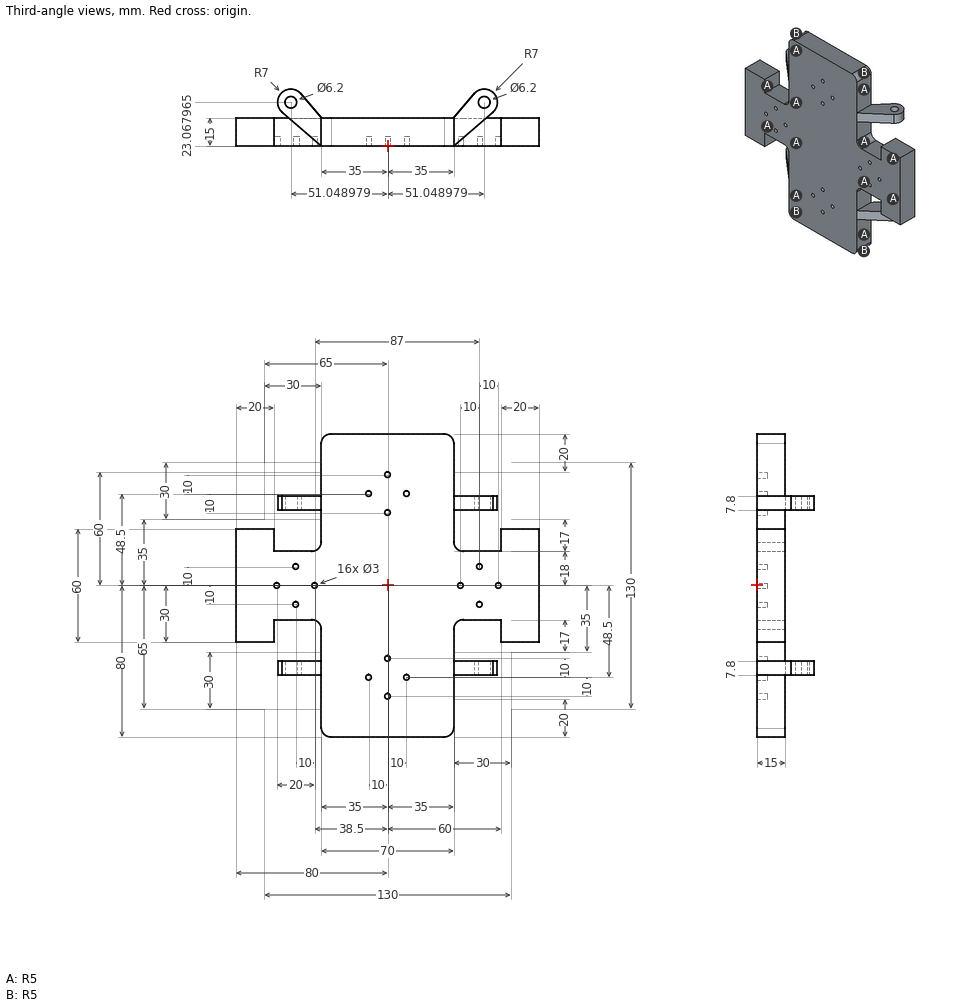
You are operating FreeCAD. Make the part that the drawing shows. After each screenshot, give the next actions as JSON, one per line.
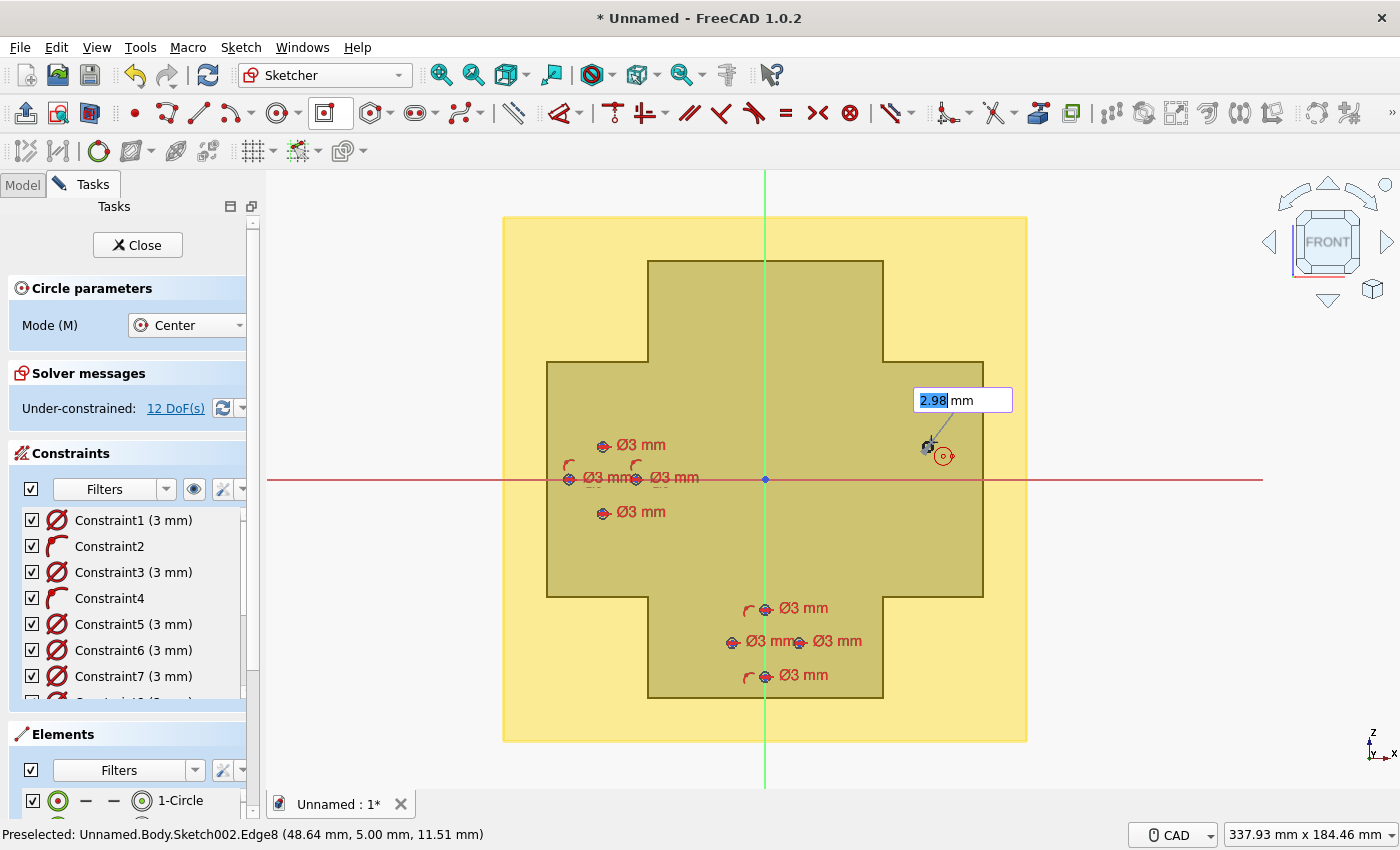
{"action": "type", "text": "3"}
{"action": "key", "text": "Return"}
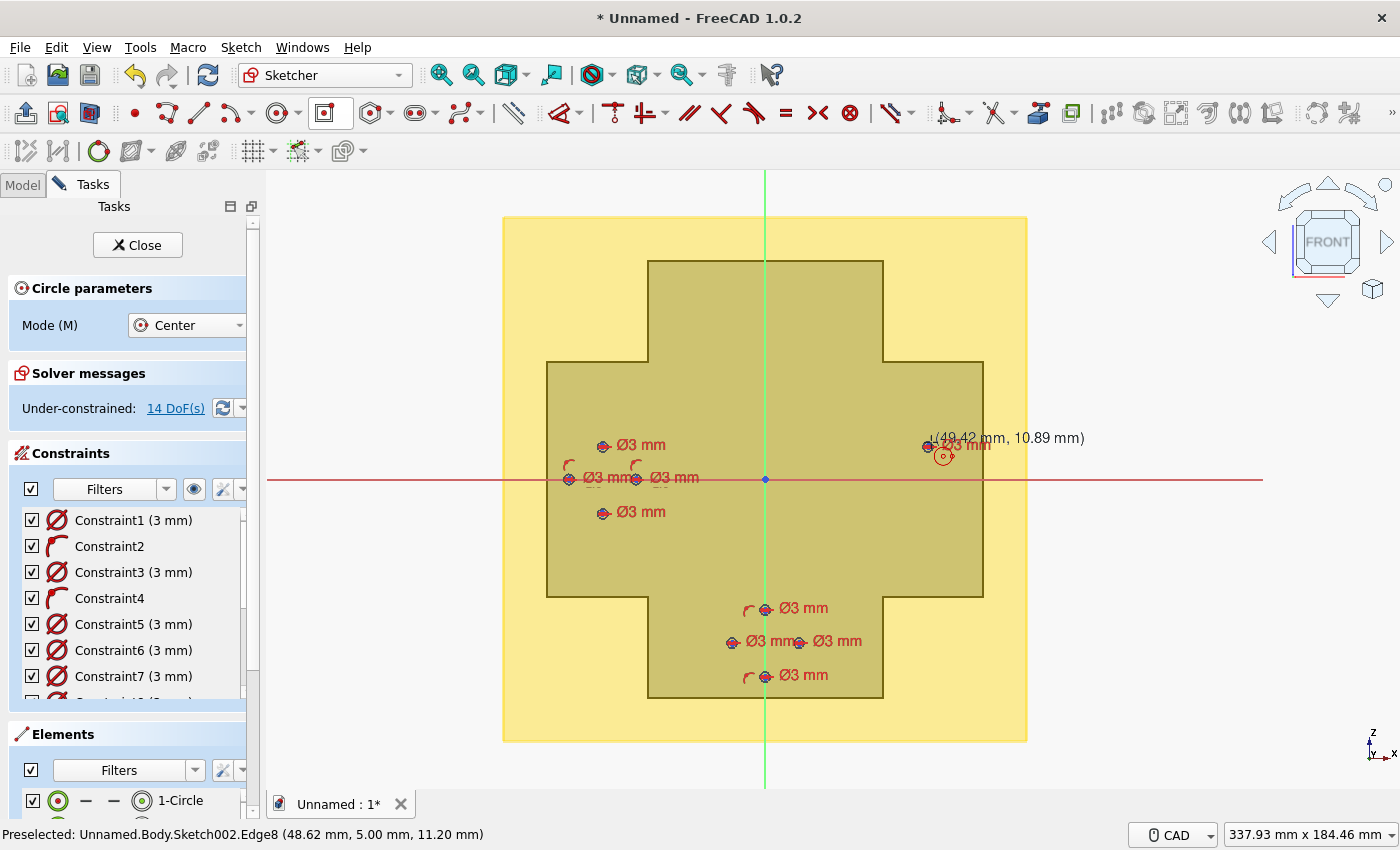
{"action": "scroll", "coordinate": [894, 480], "scroll_direction": "up", "scroll_amount": 8}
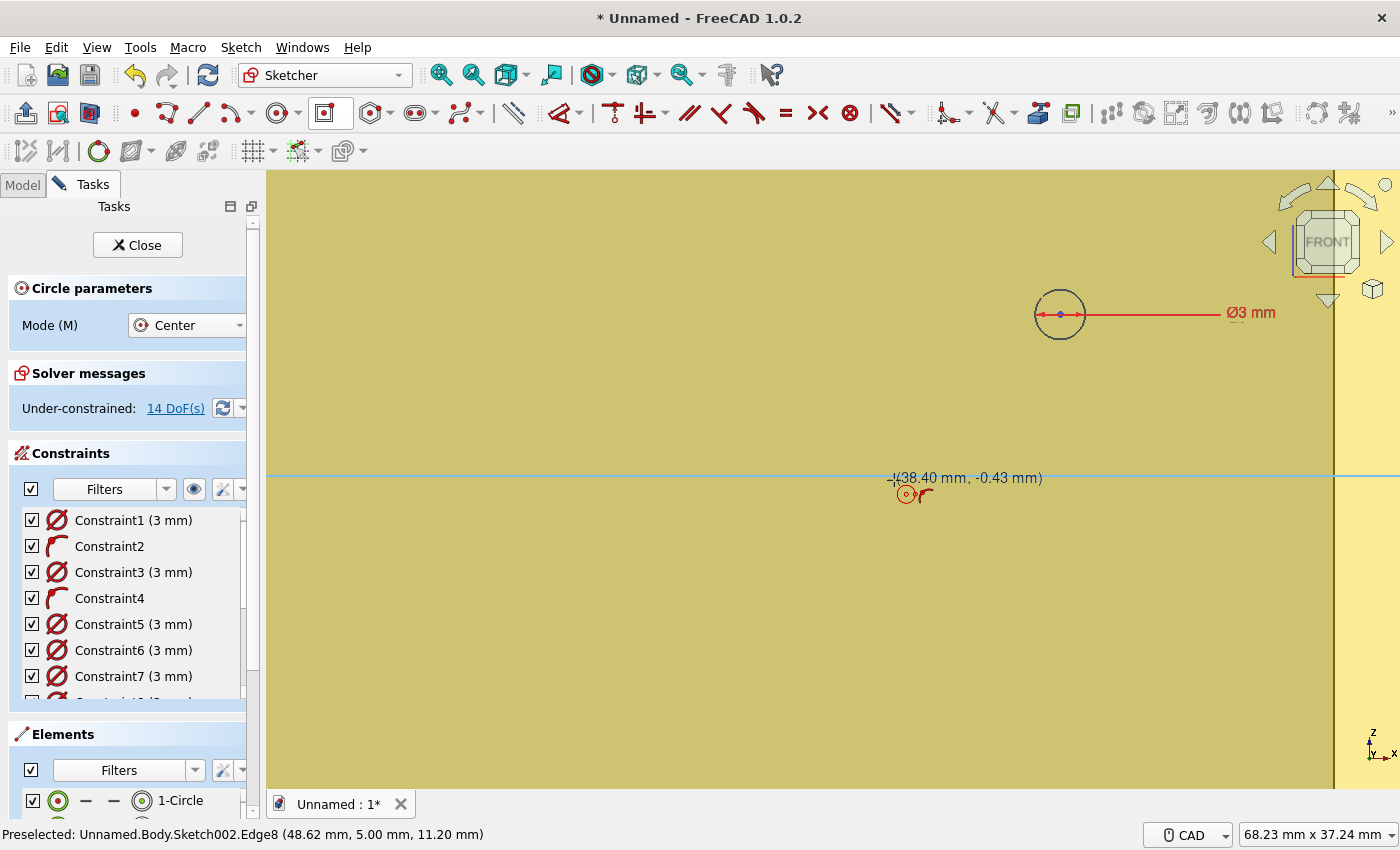
{"action": "scroll", "coordinate": [894, 480], "scroll_direction": "down", "scroll_amount": 8}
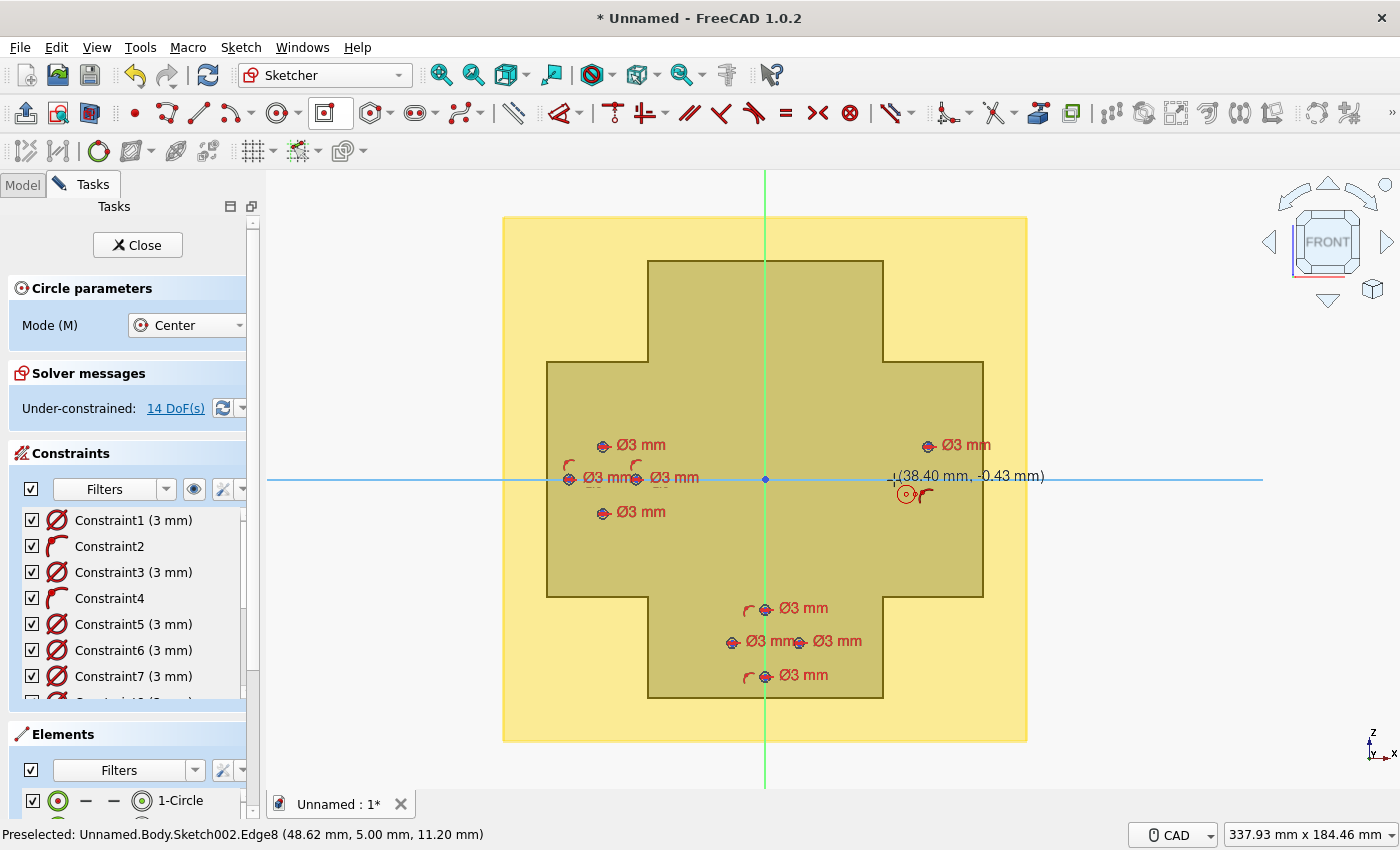
{"action": "left_click", "coordinate": [894, 480]}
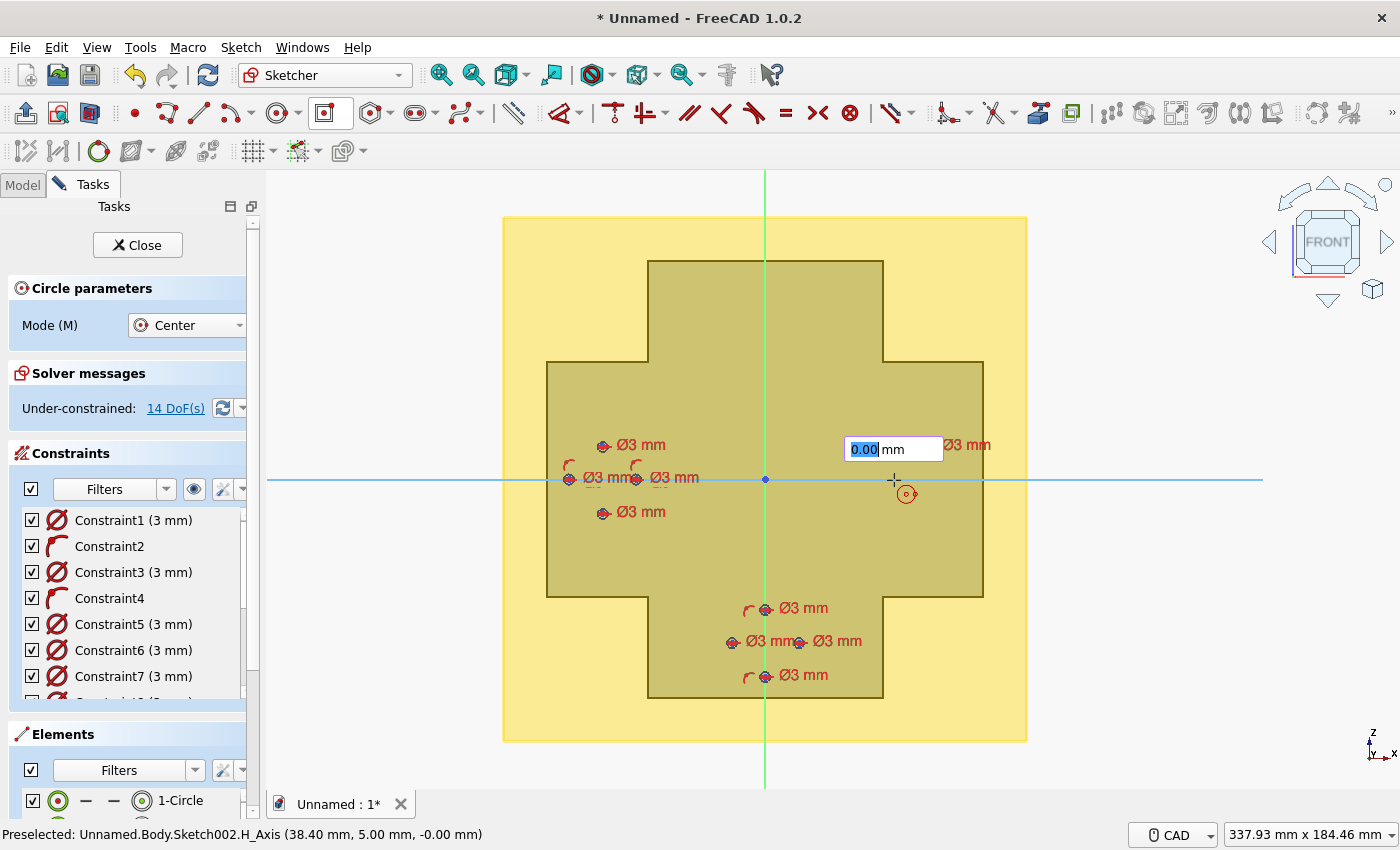
{"action": "scroll", "coordinate": [893, 484], "scroll_direction": "up", "scroll_amount": 7}
{"action": "mouse_move", "coordinate": [890, 484]}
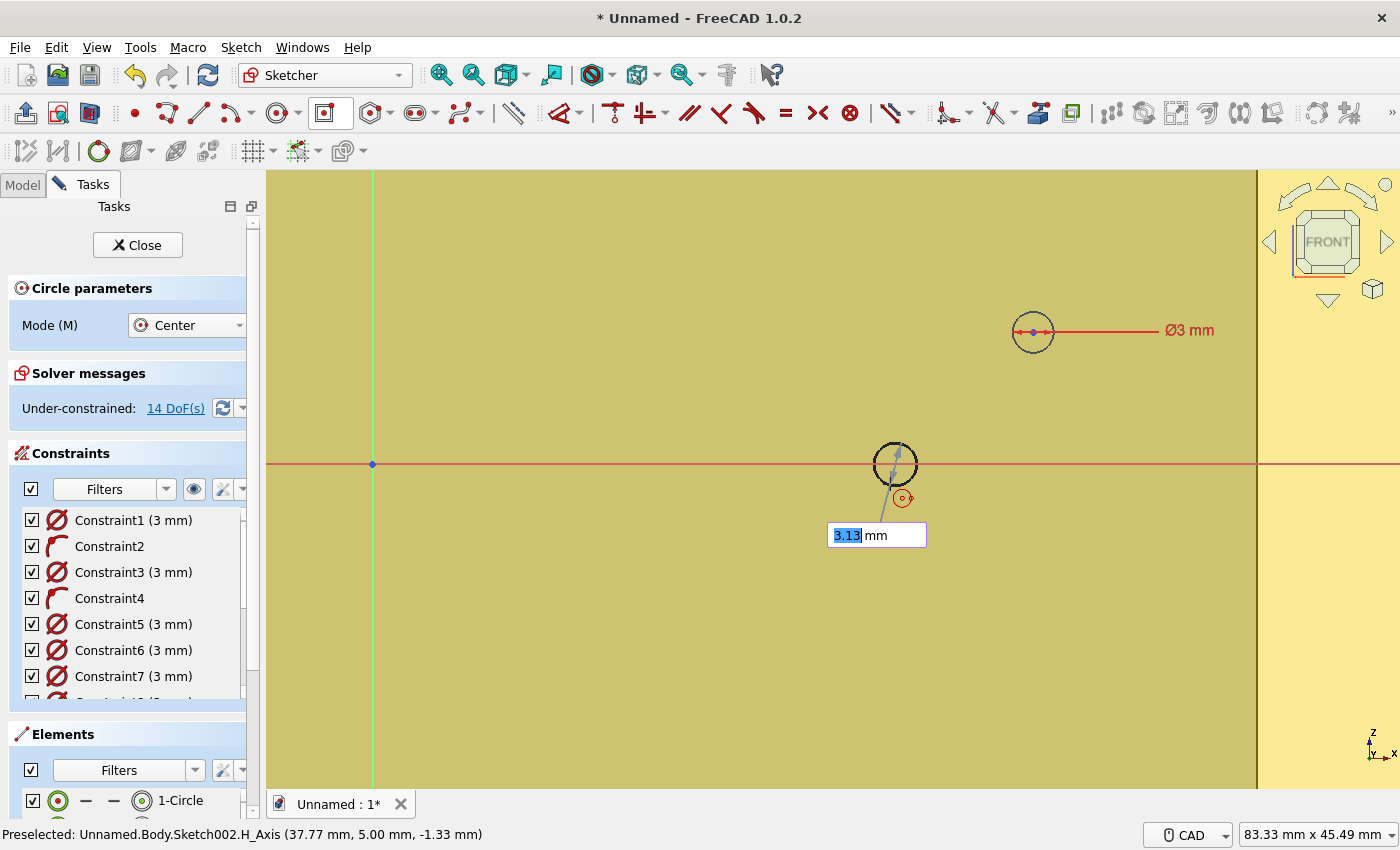
{"action": "type", "text": "3"}
{"action": "key", "text": "Return"}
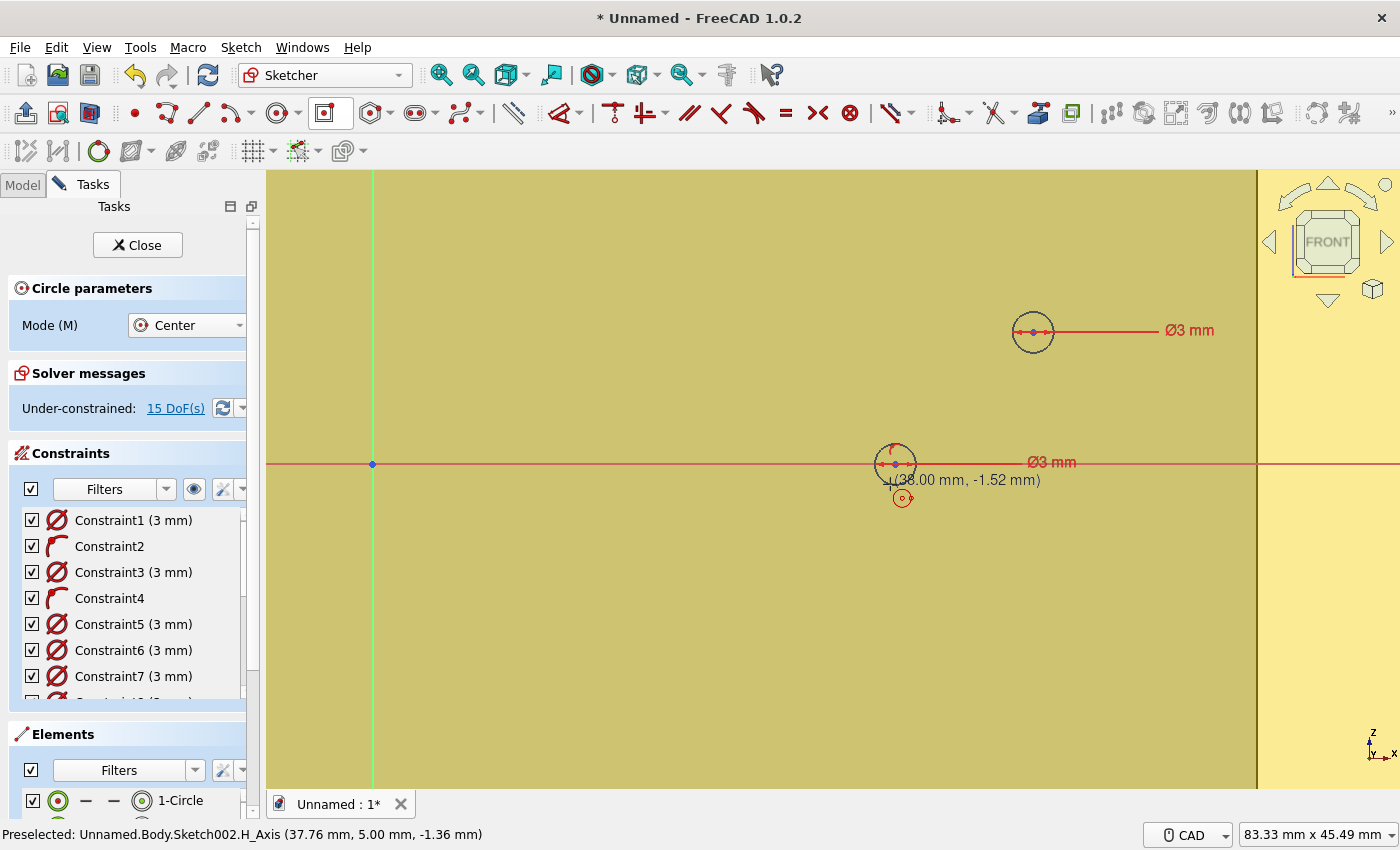
{"action": "scroll", "coordinate": [893, 484], "scroll_direction": "down", "scroll_amount": 7}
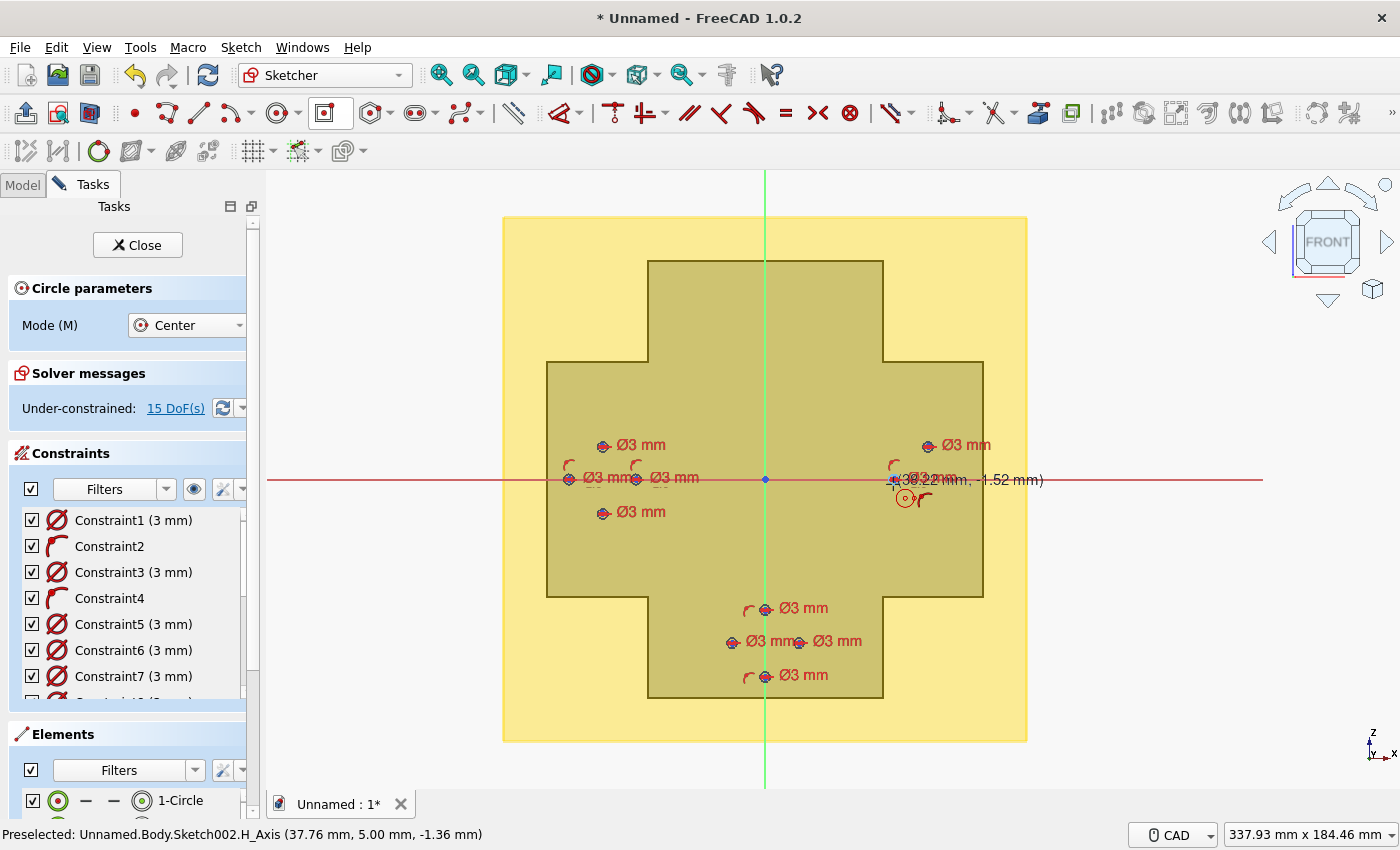
{"action": "left_click", "coordinate": [928, 513]}
{"action": "mouse_move", "coordinate": [931, 510]}